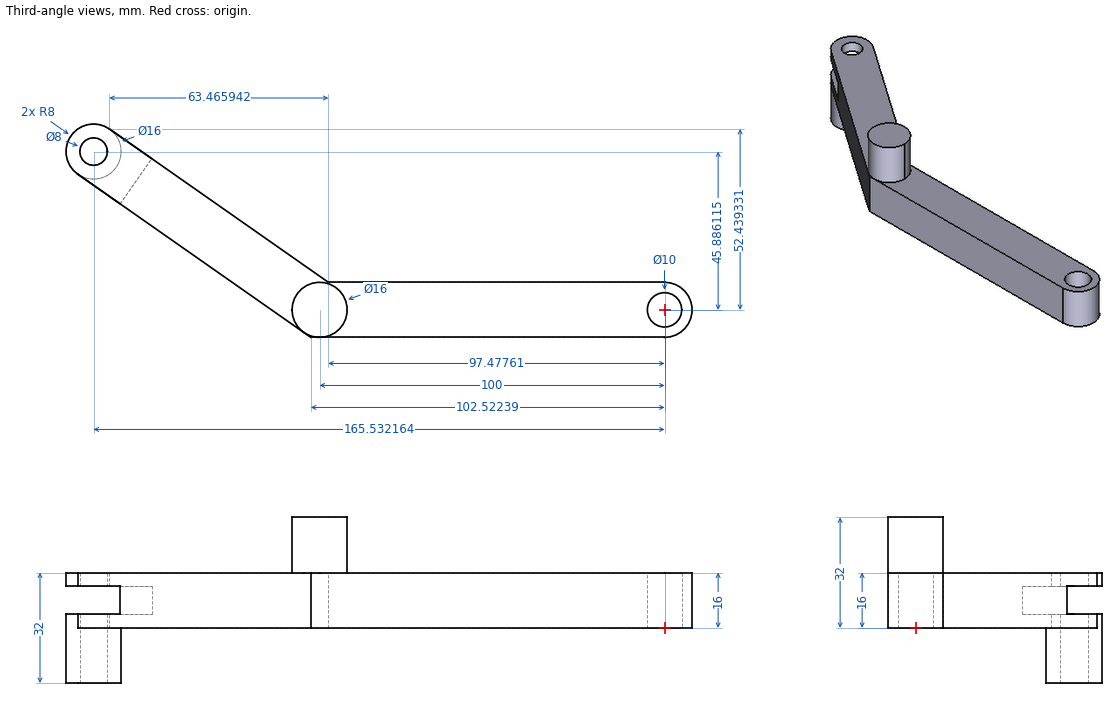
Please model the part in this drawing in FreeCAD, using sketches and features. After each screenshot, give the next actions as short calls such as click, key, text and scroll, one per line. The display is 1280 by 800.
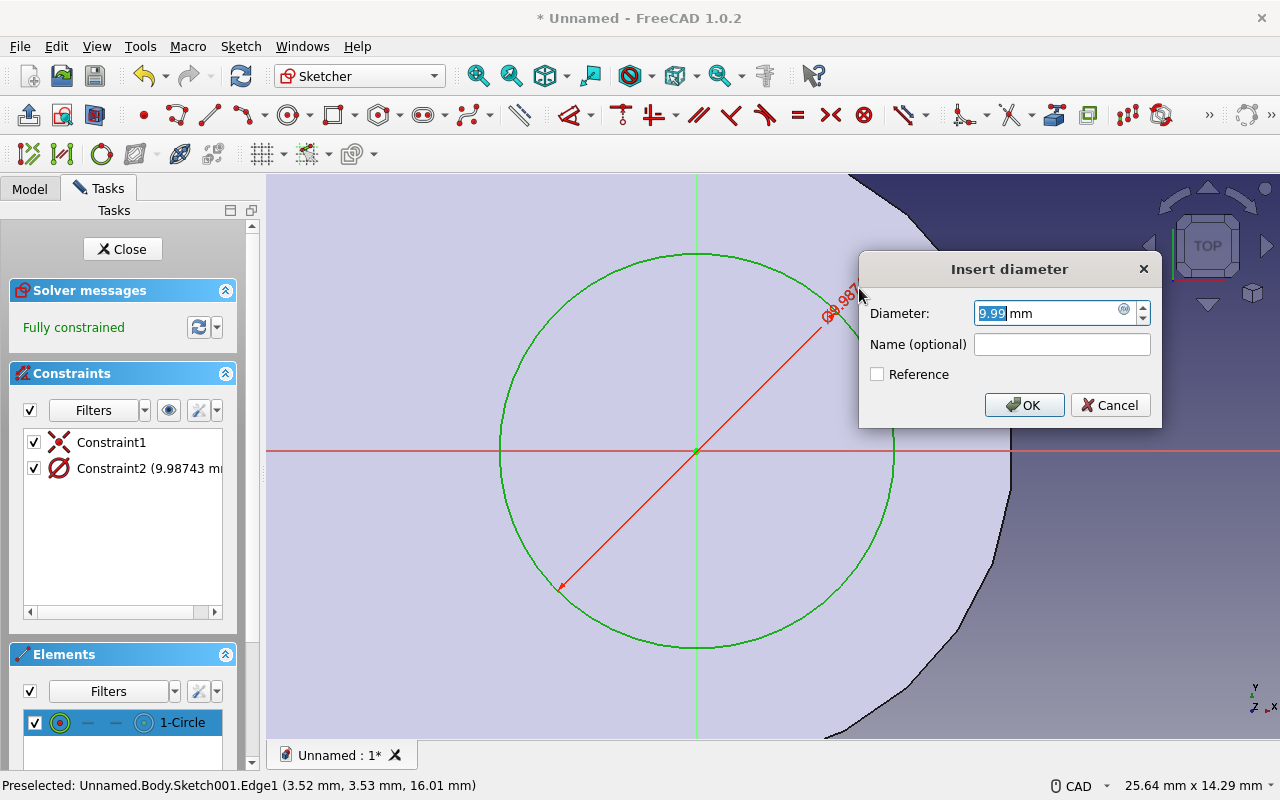
text(10)
key(Return)
key(Escape)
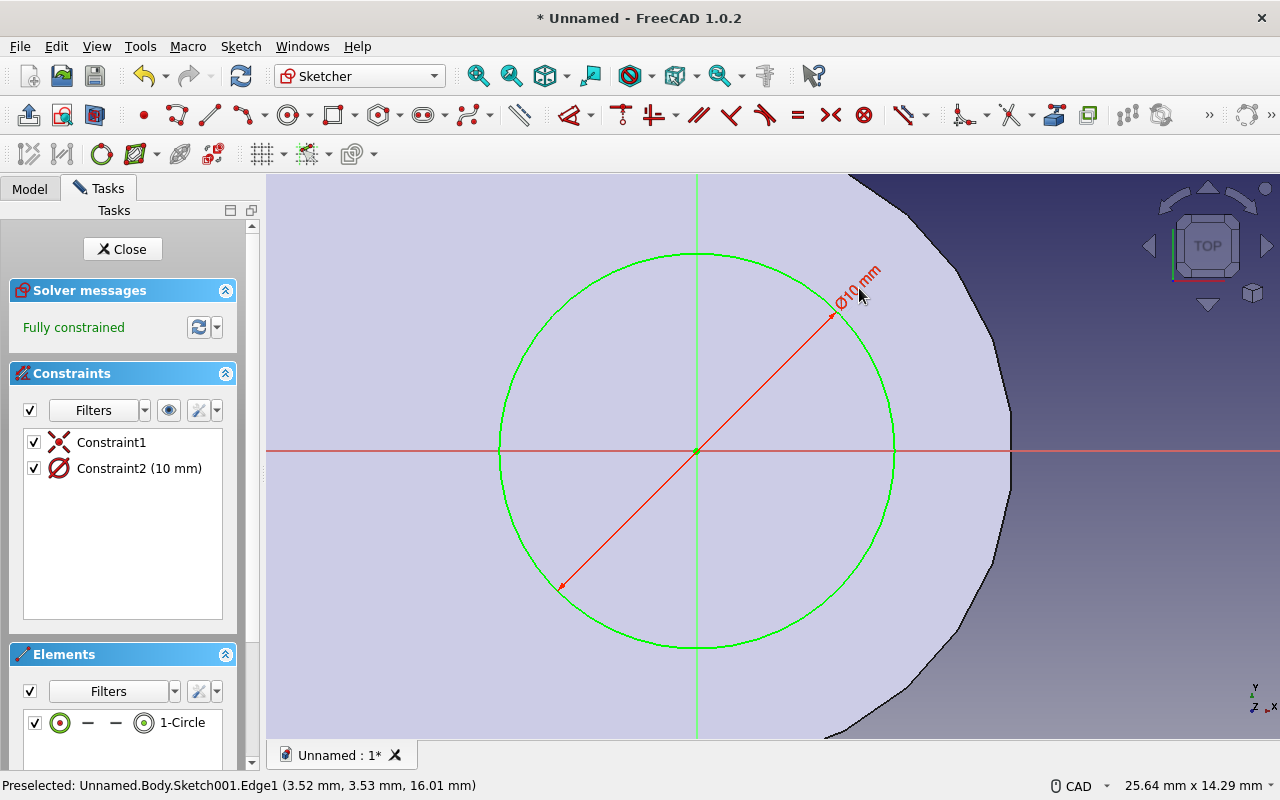
click(123, 249)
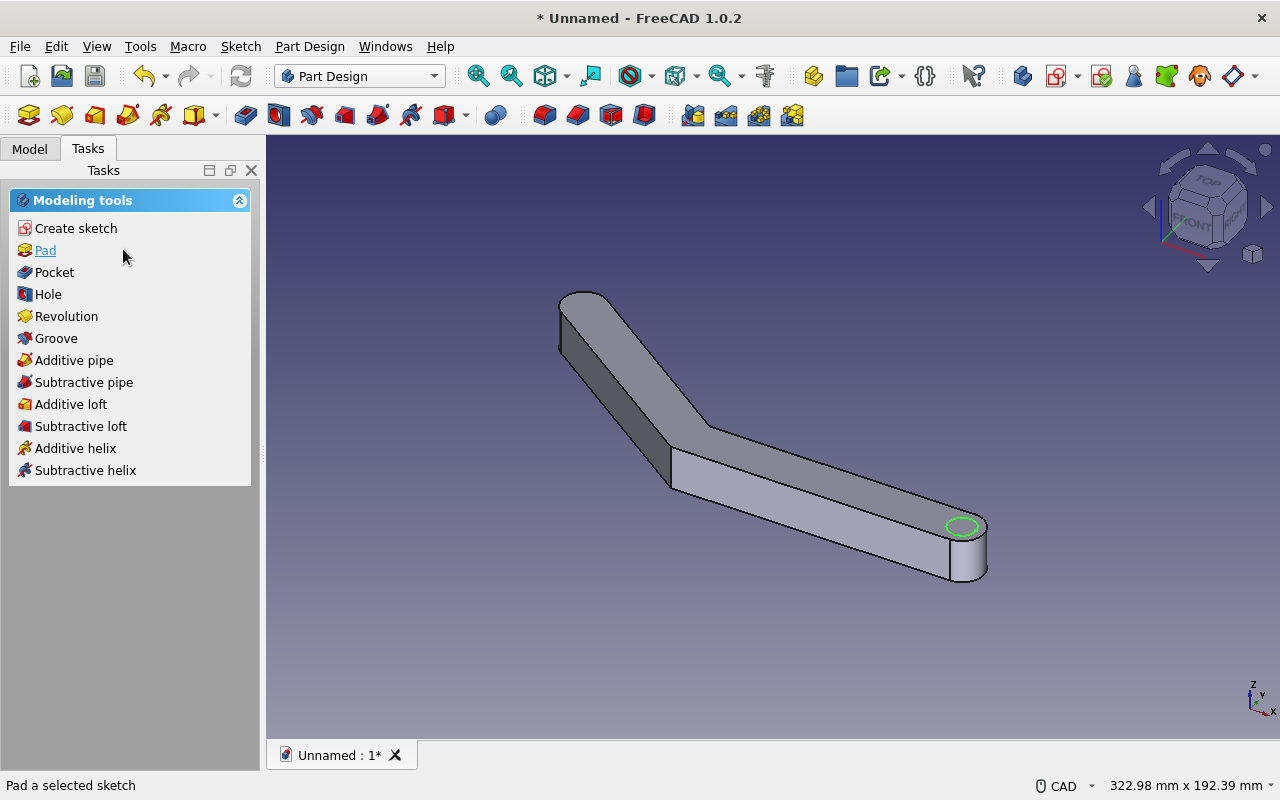
click(246, 116)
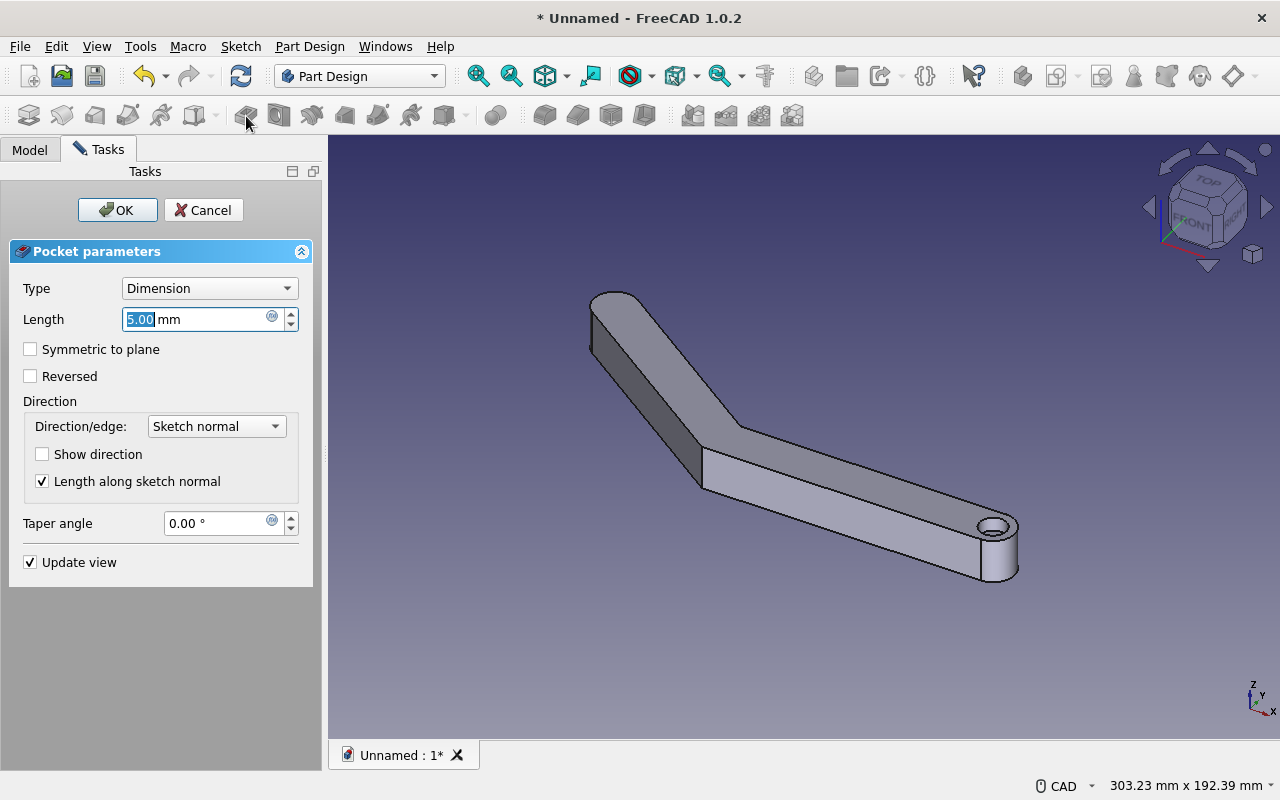
text(16)
key(Tab)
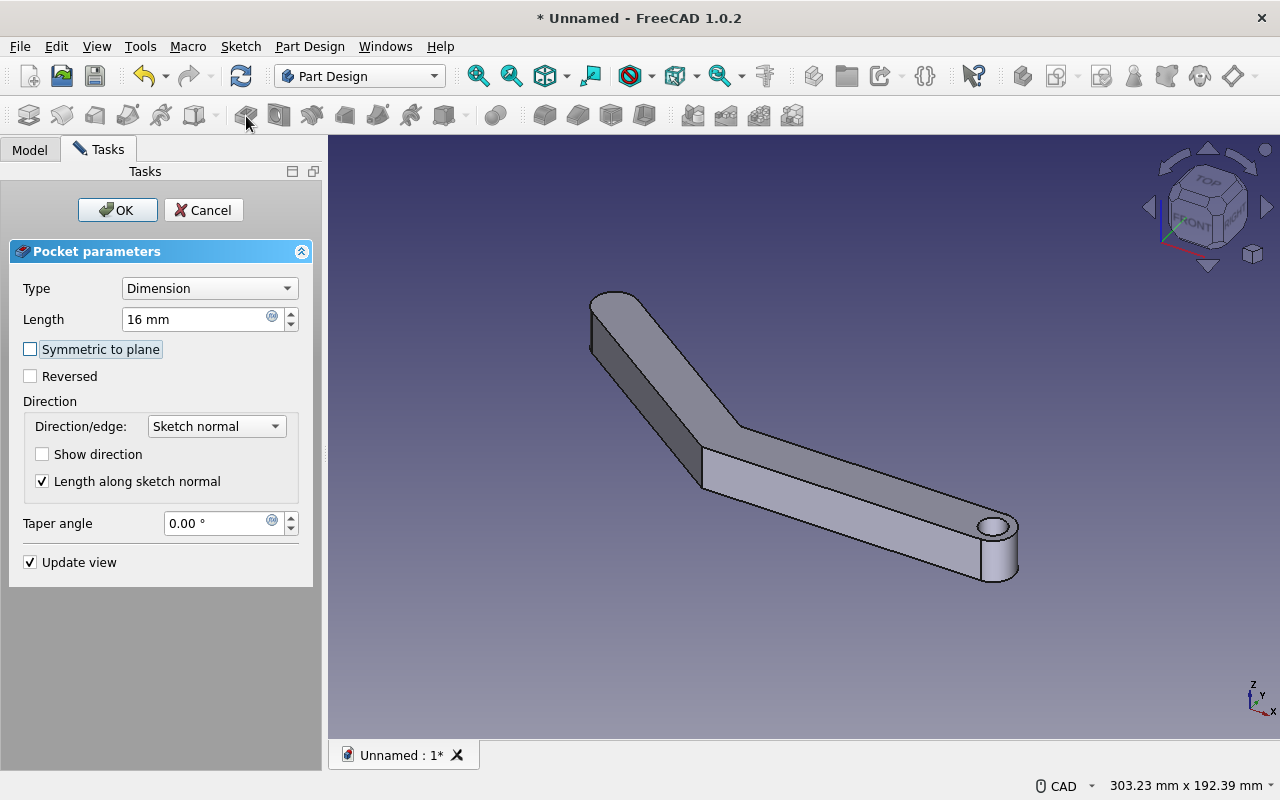
click(118, 210)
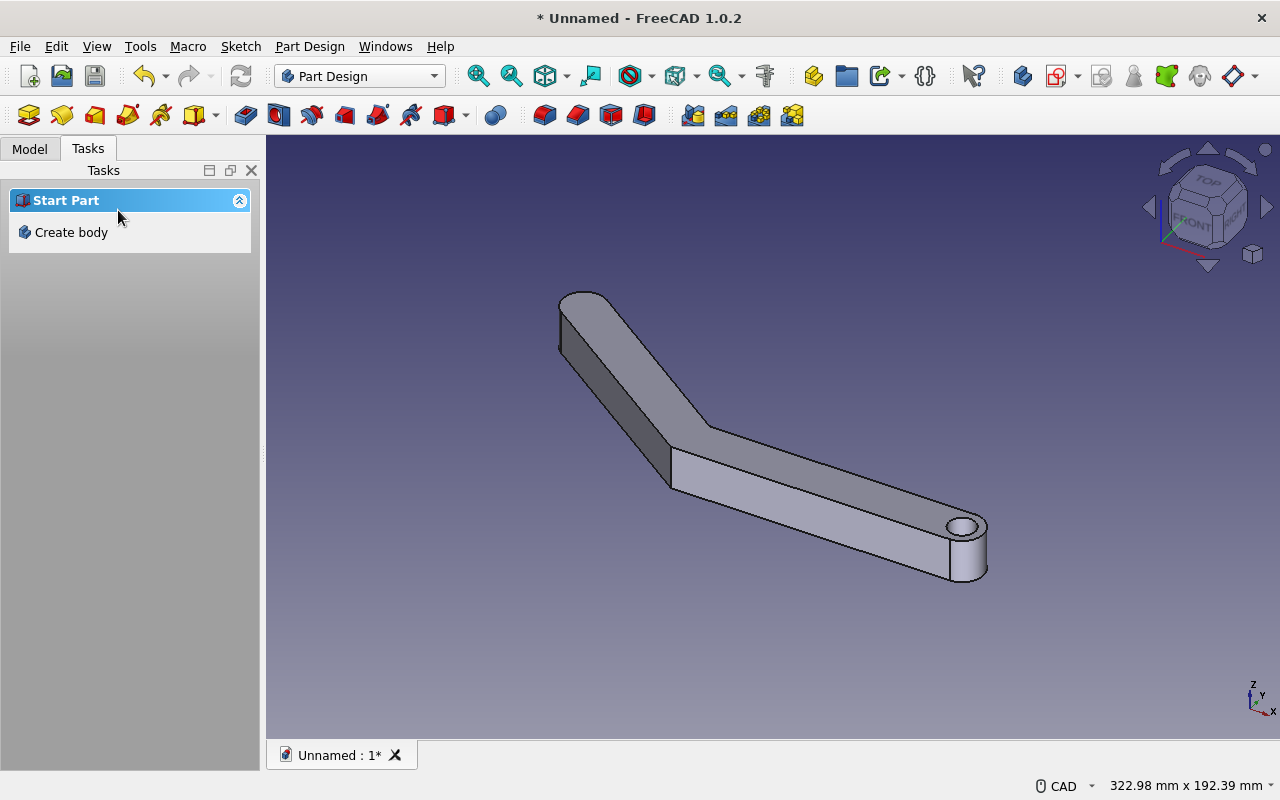
click(1056, 76)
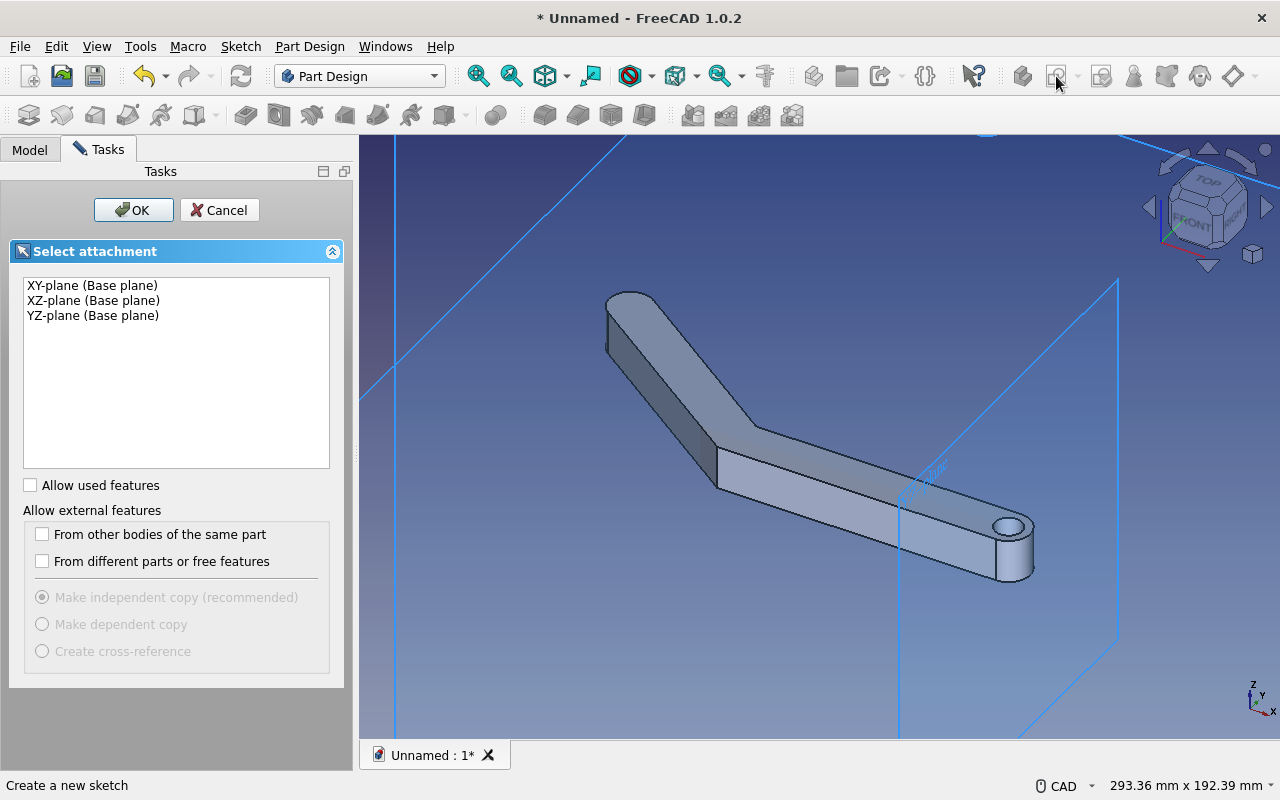
click(84, 286)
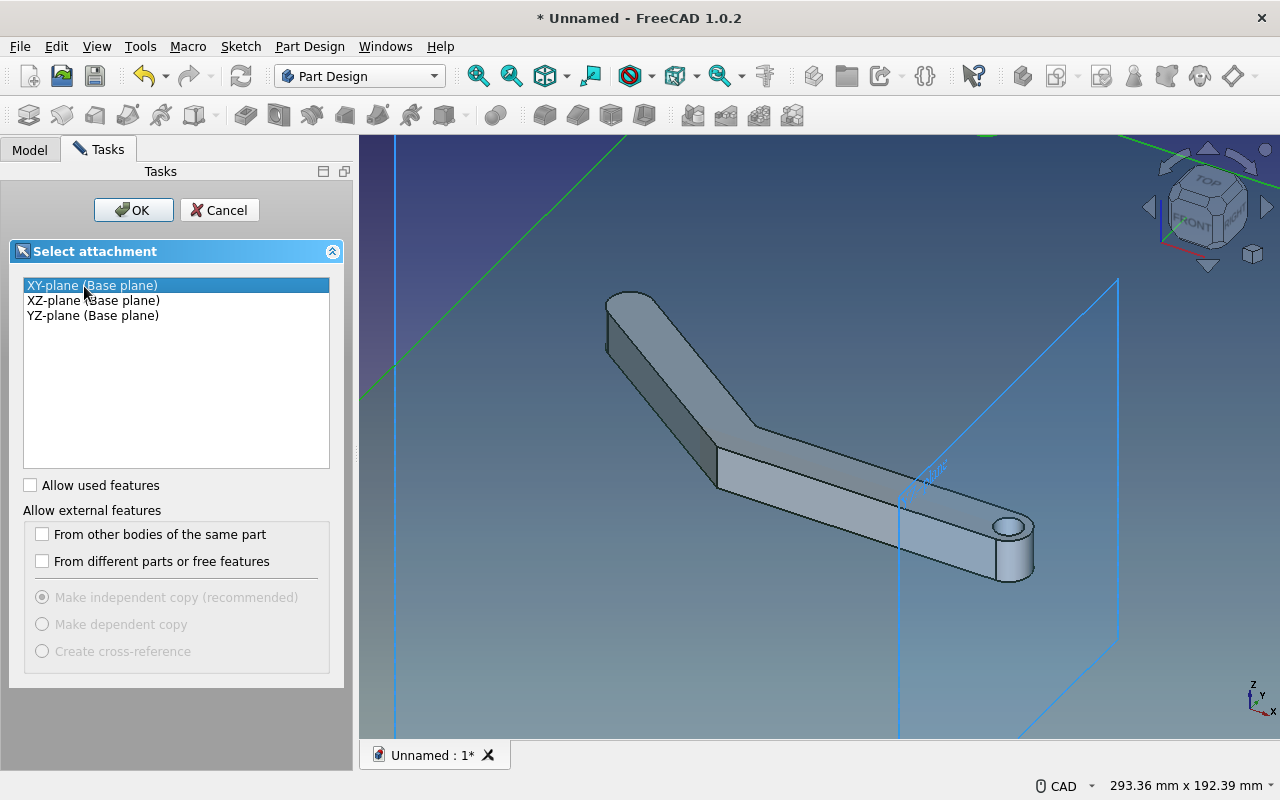
click(134, 210)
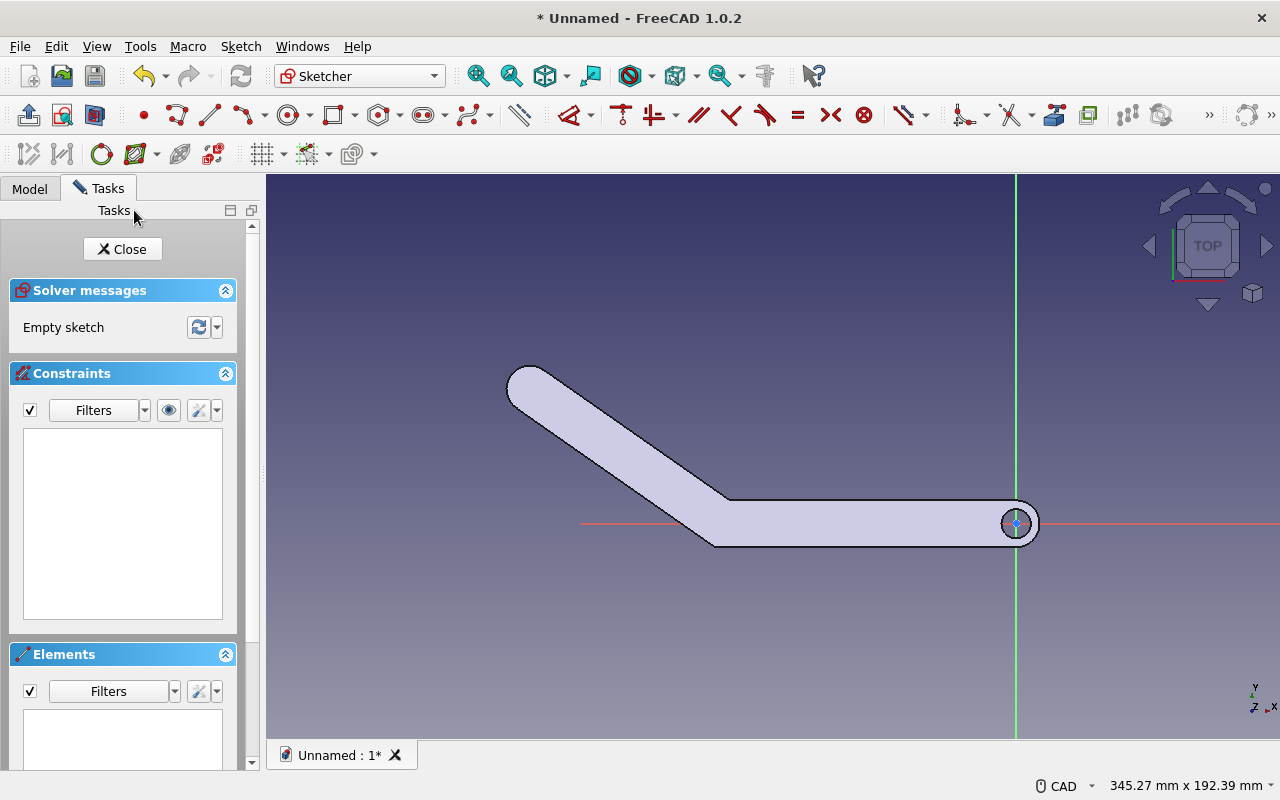
click(95, 116)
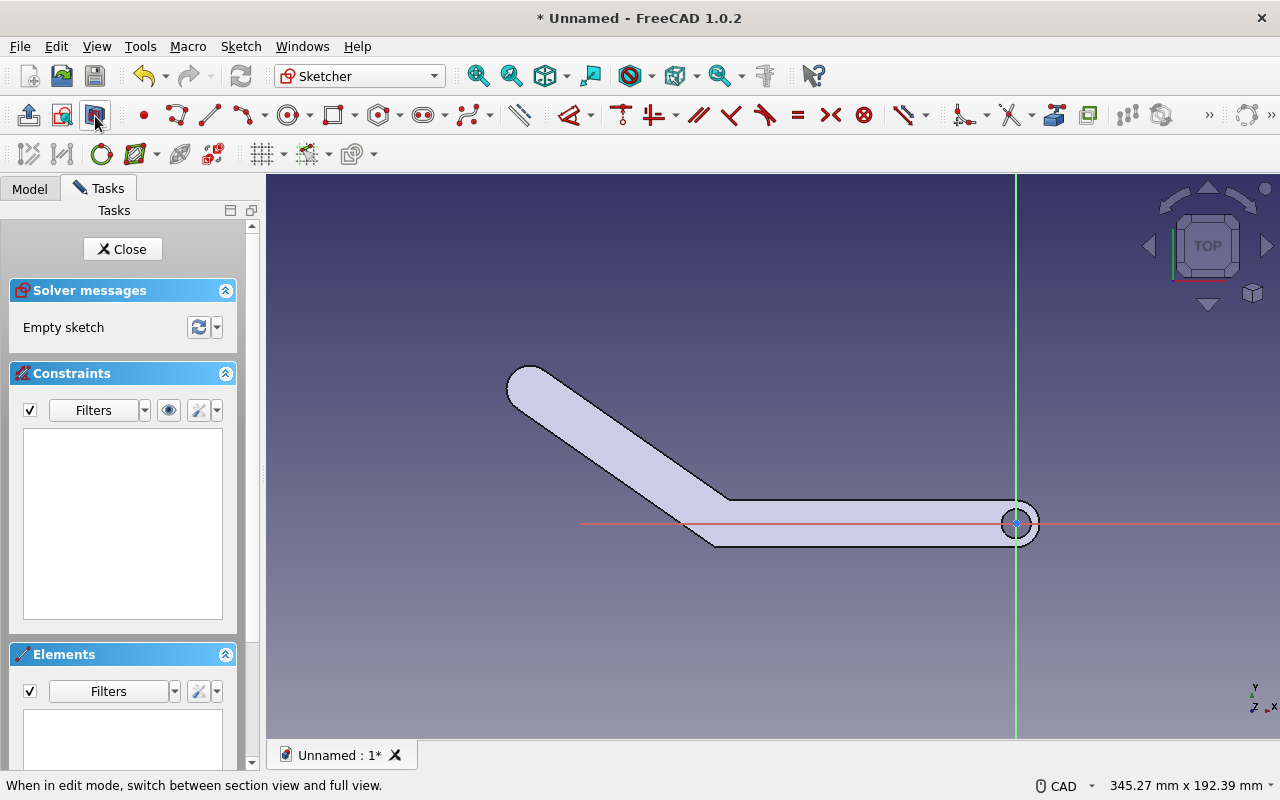
scroll(725, 534, up, 10)